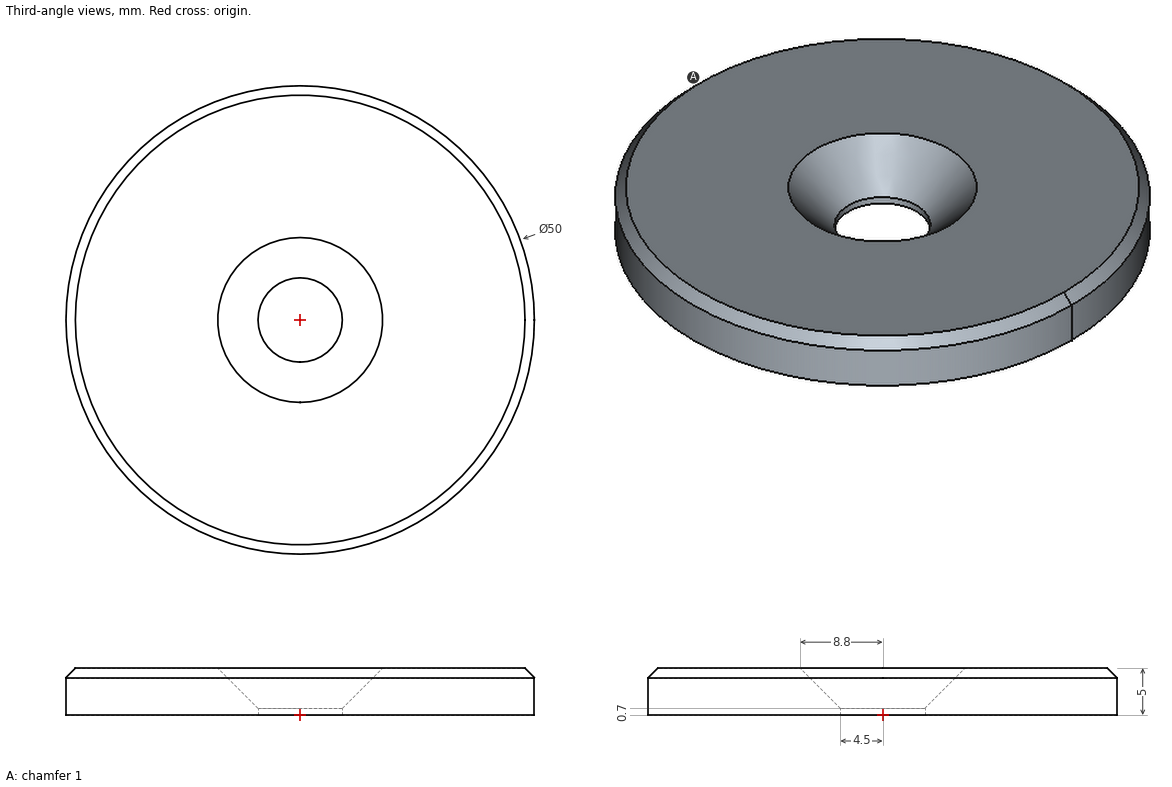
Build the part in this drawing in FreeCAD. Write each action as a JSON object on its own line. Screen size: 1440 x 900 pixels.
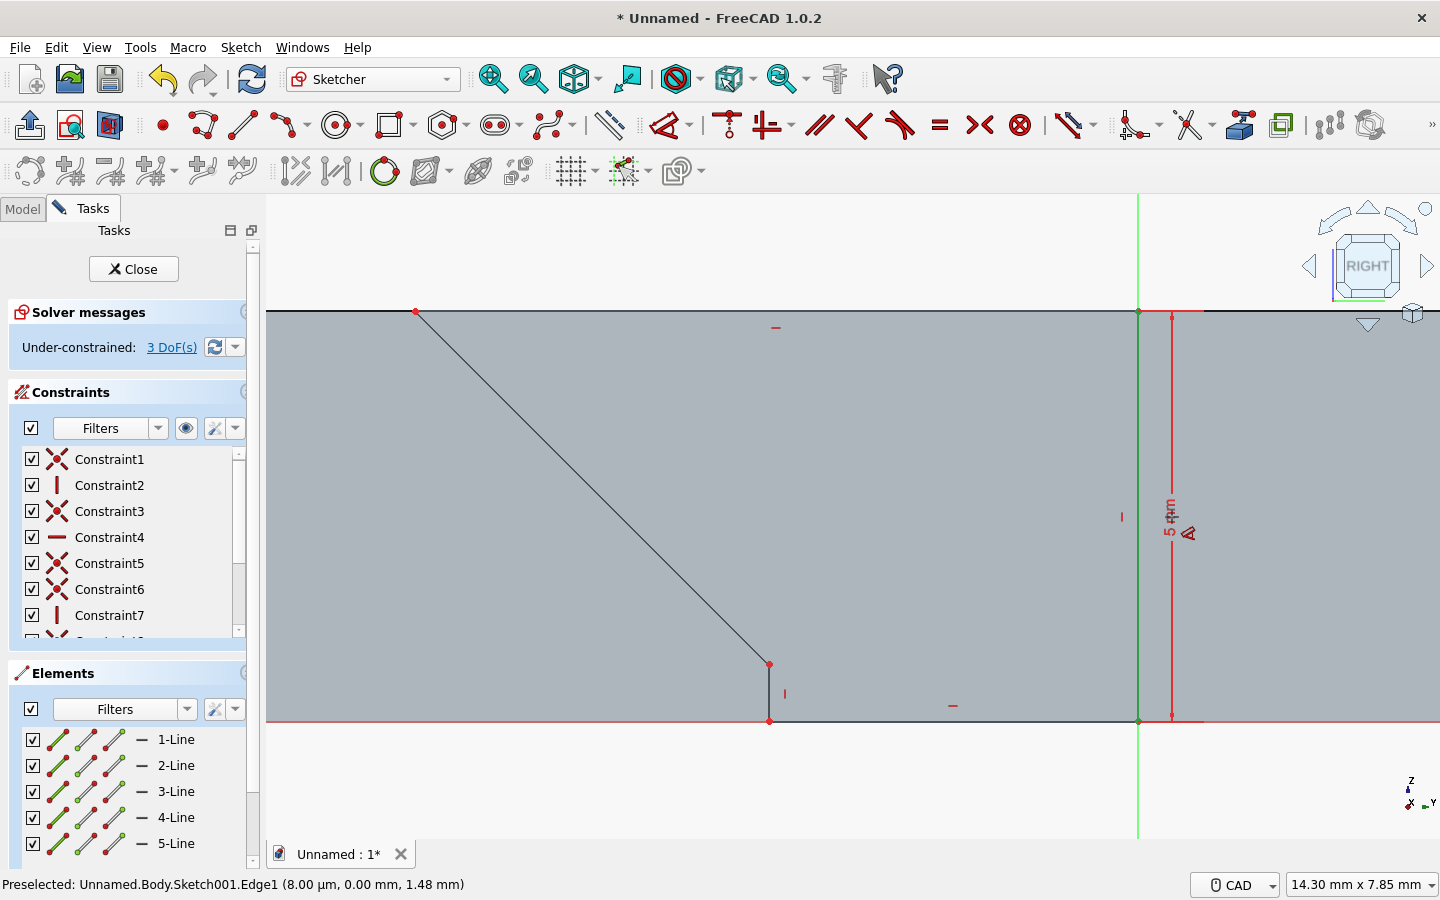
{"action": "left_click", "coordinate": [921, 311]}
{"action": "left_click", "coordinate": [777, 277]}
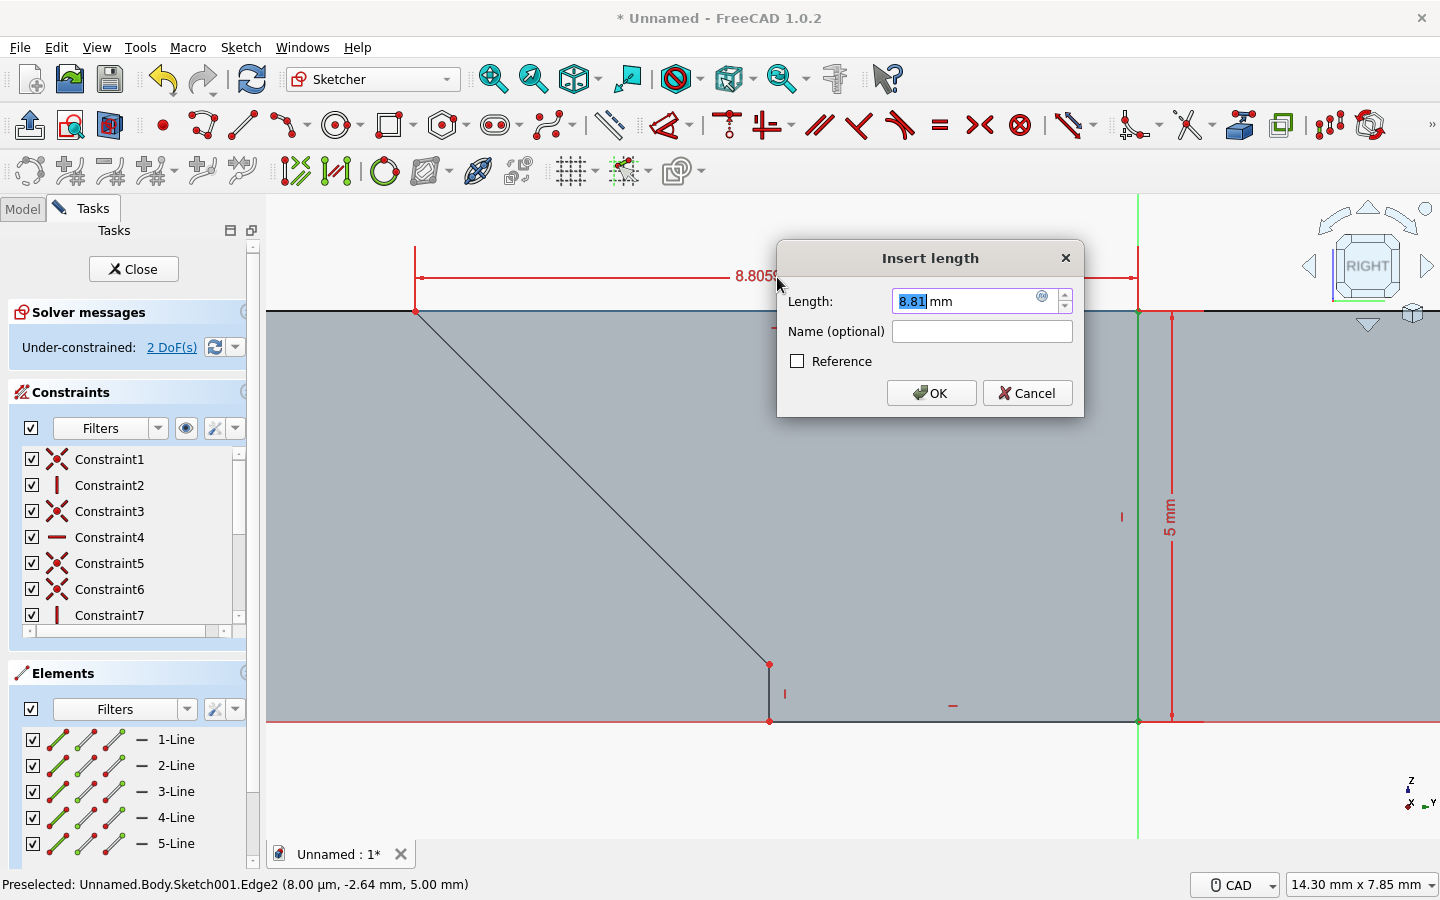
{"action": "type", "text": "8.8"}
{"action": "key", "text": "Return"}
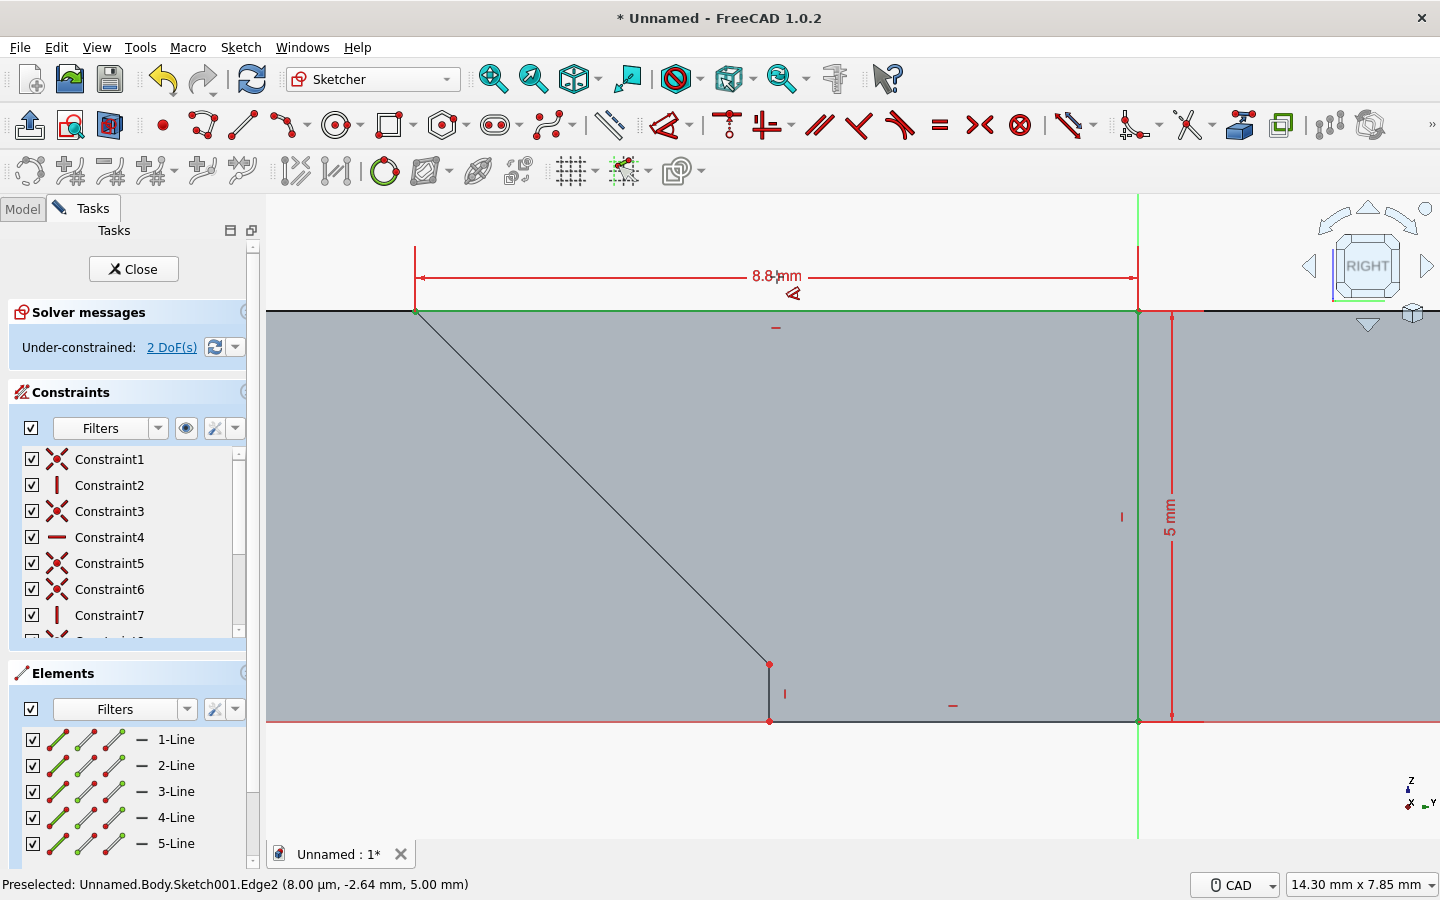
{"action": "left_click", "coordinate": [769, 682]}
{"action": "left_click", "coordinate": [735, 693]}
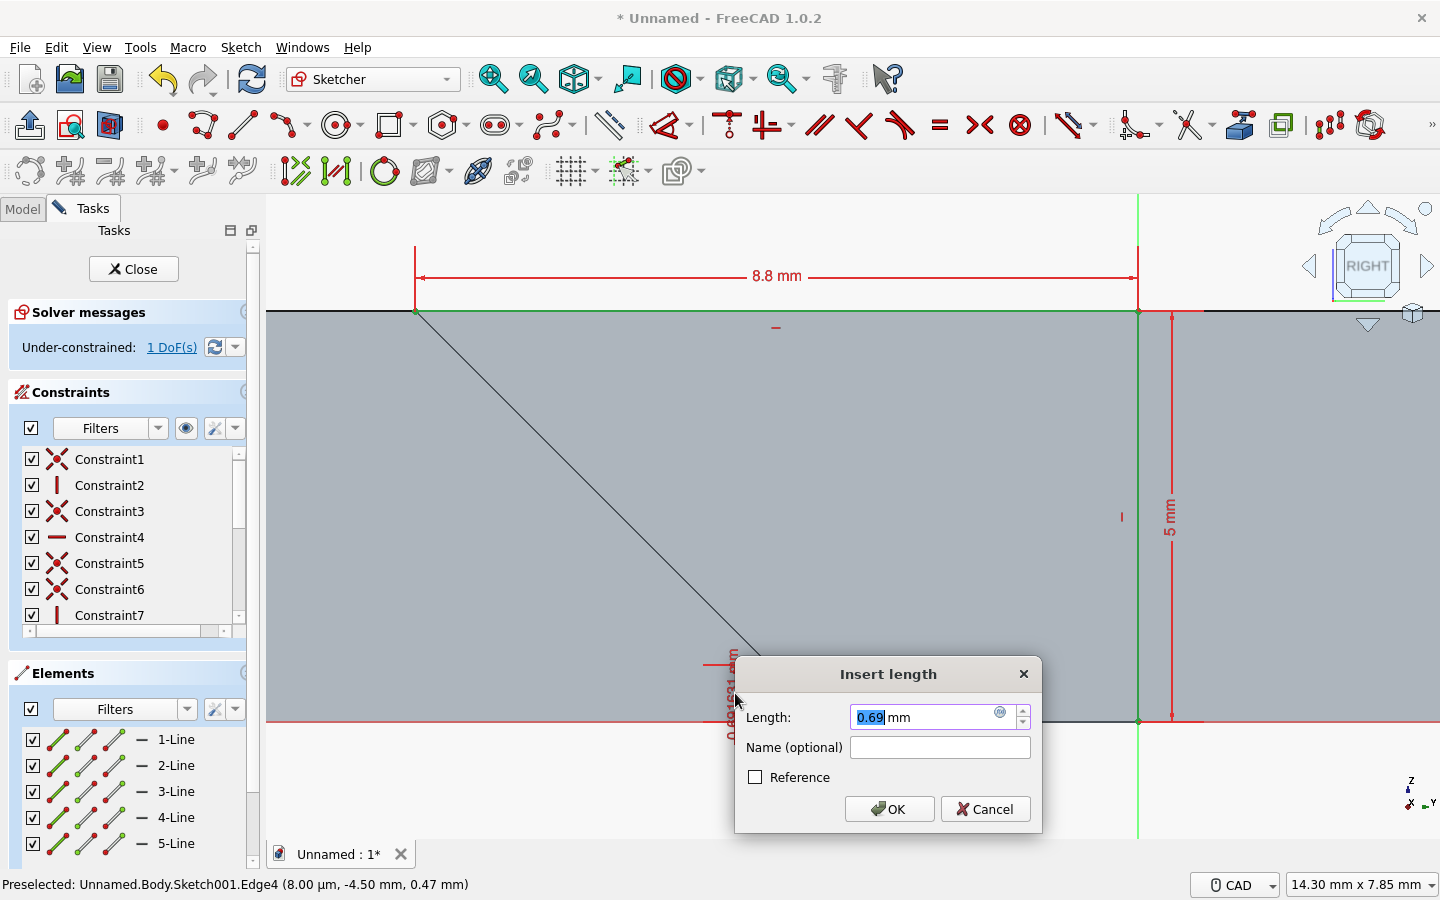
{"action": "type", "text": "0.7"}
{"action": "key", "text": "Return"}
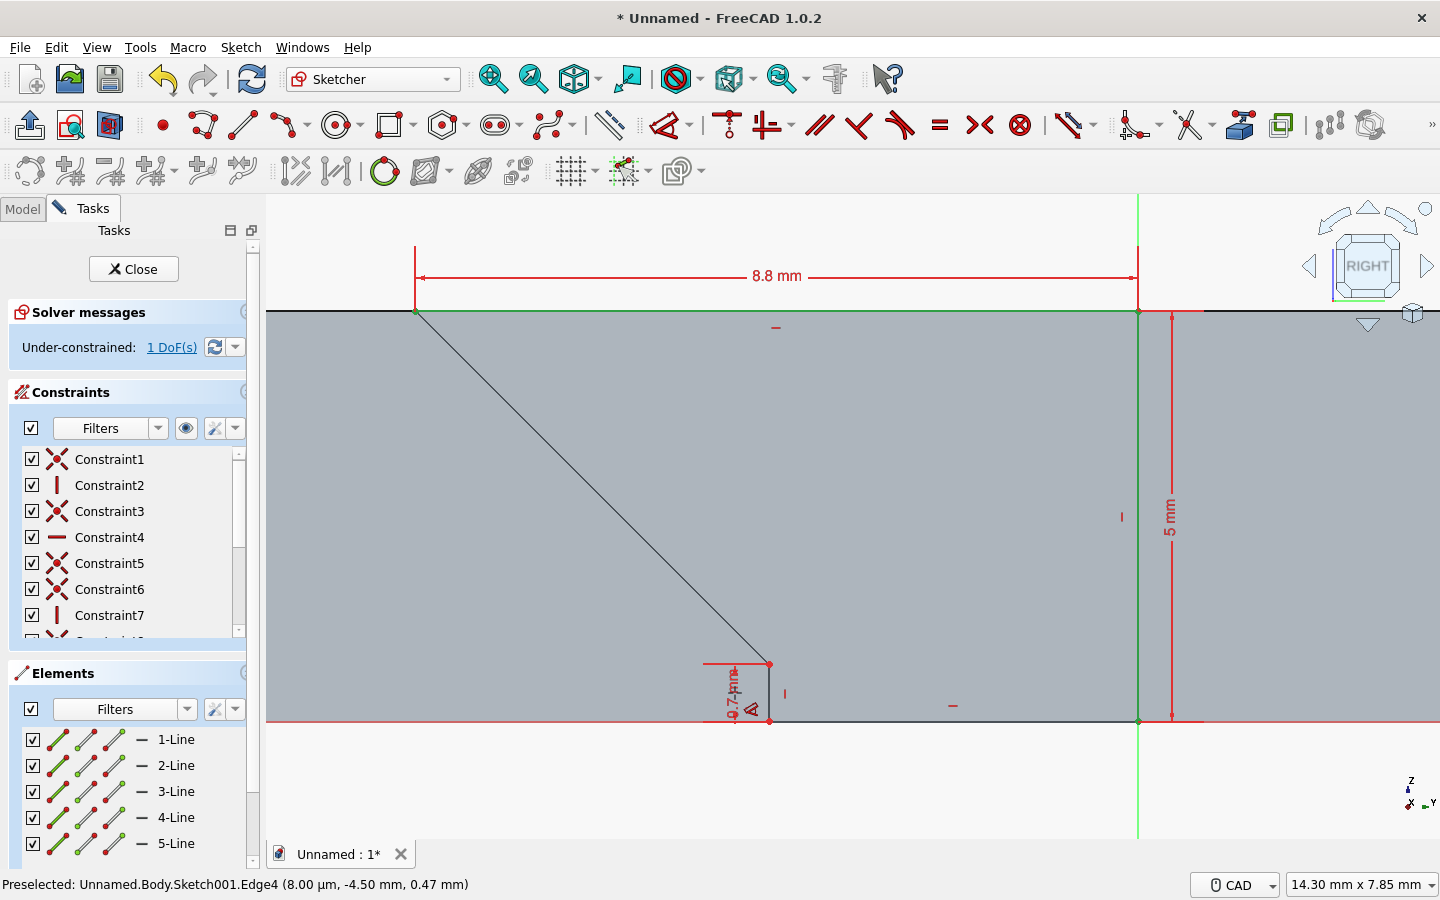
{"action": "left_click", "coordinate": [880, 722]}
{"action": "left_click", "coordinate": [954, 756]}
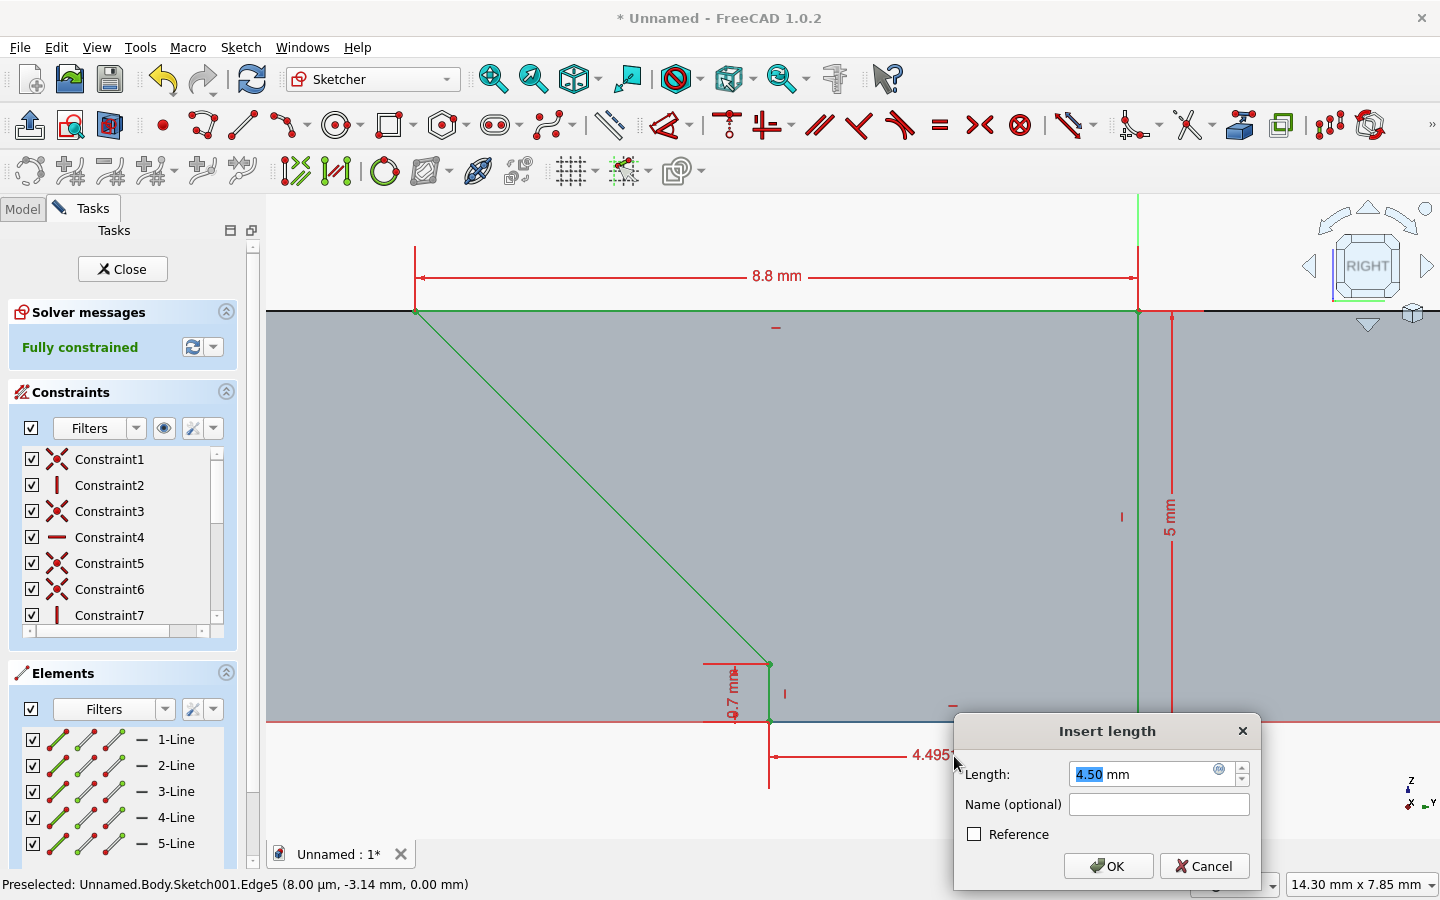
{"action": "type", "text": "4.5"}
{"action": "key", "text": "Return"}
{"action": "key", "text": "Escape"}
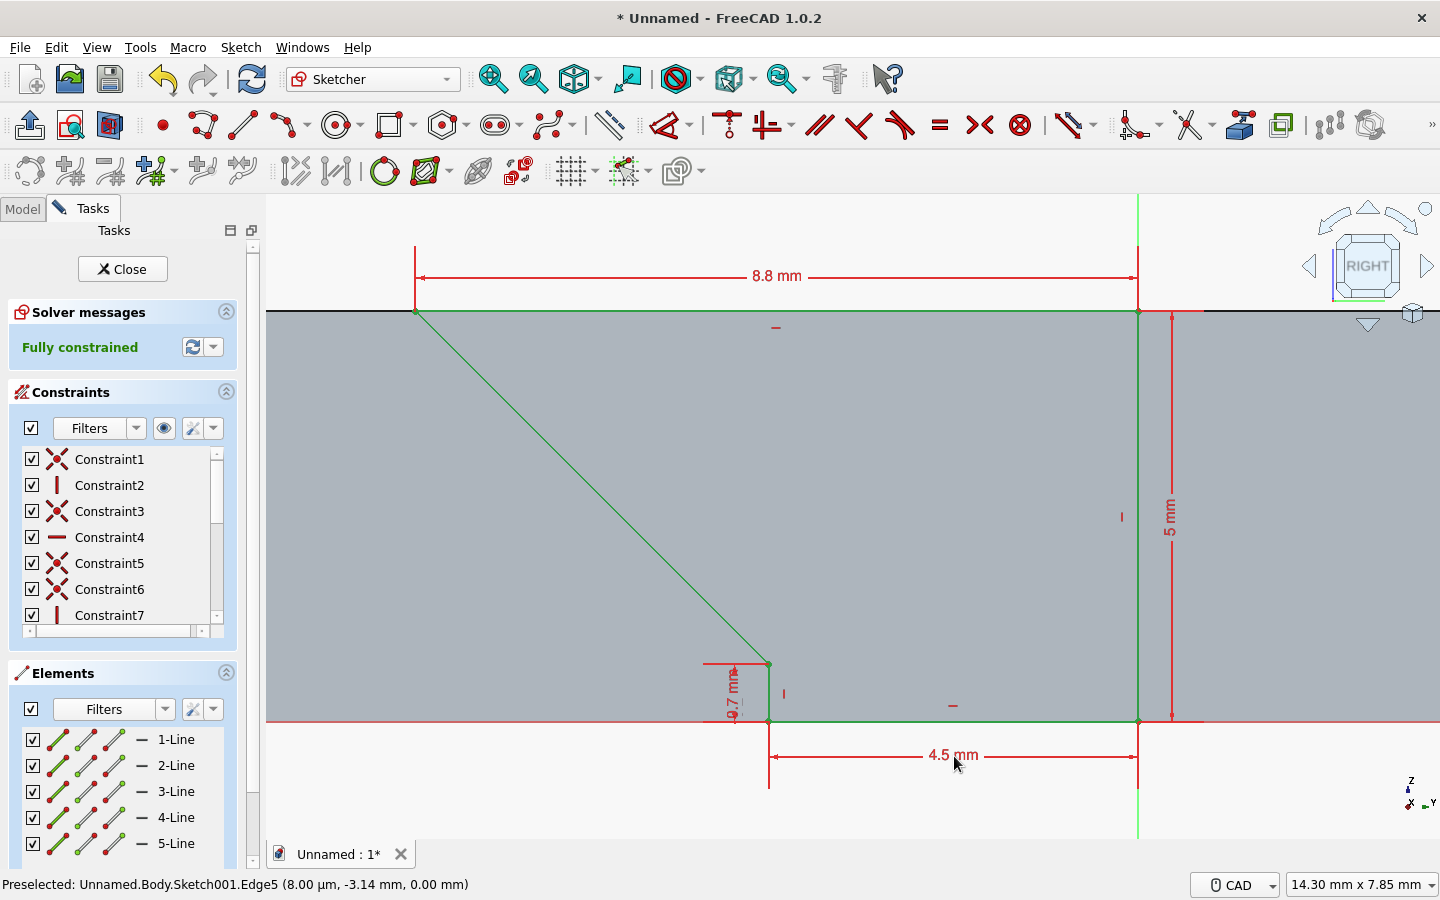
{"action": "left_click", "coordinate": [123, 269]}